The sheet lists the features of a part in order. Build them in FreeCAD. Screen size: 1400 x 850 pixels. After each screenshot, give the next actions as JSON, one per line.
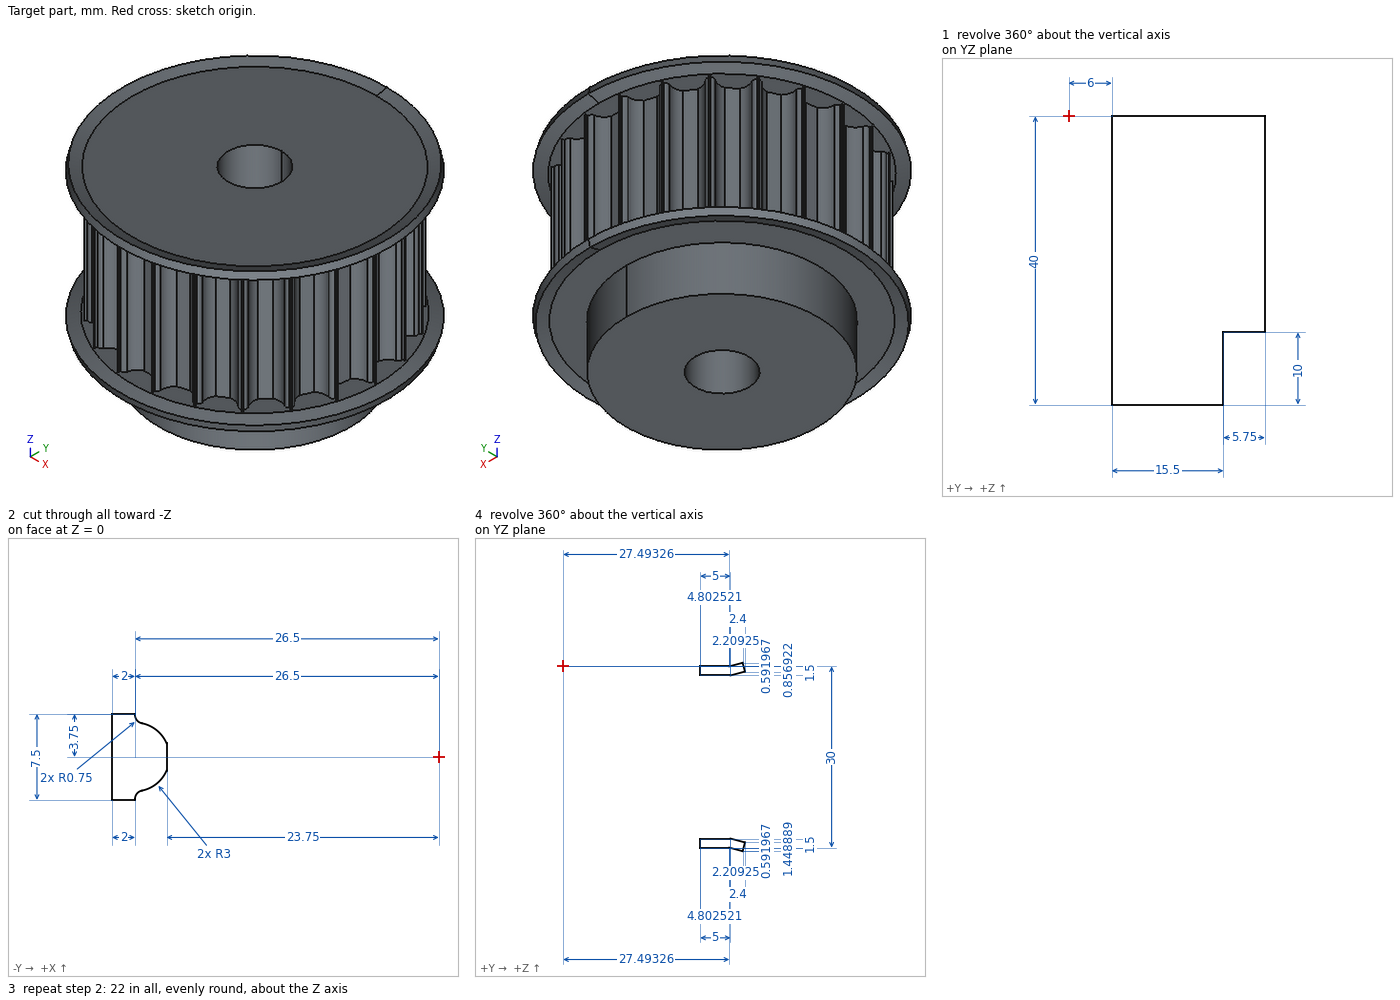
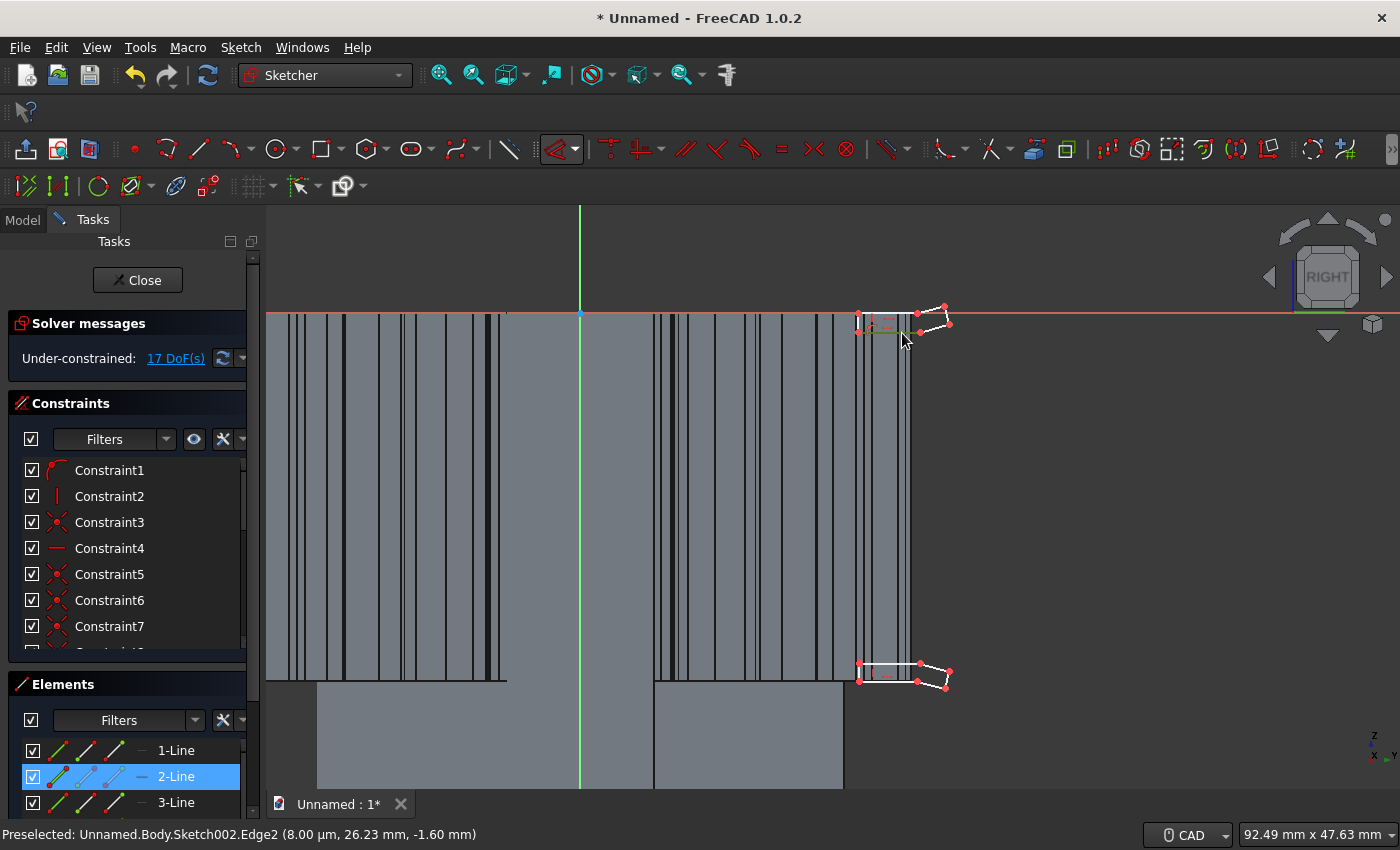
{"action": "left_click", "coordinate": [578, 150]}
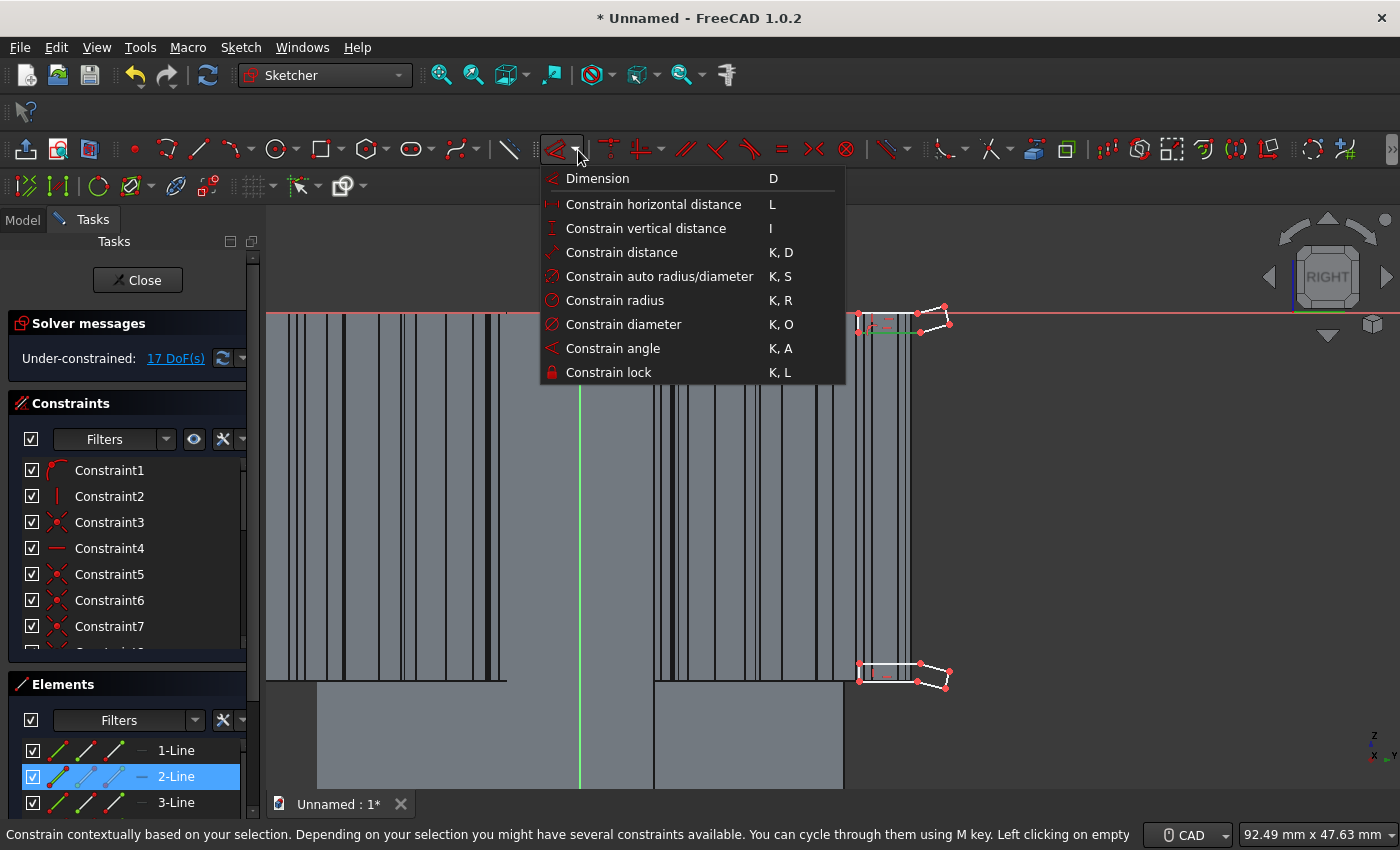
{"action": "left_click", "coordinate": [693, 204]}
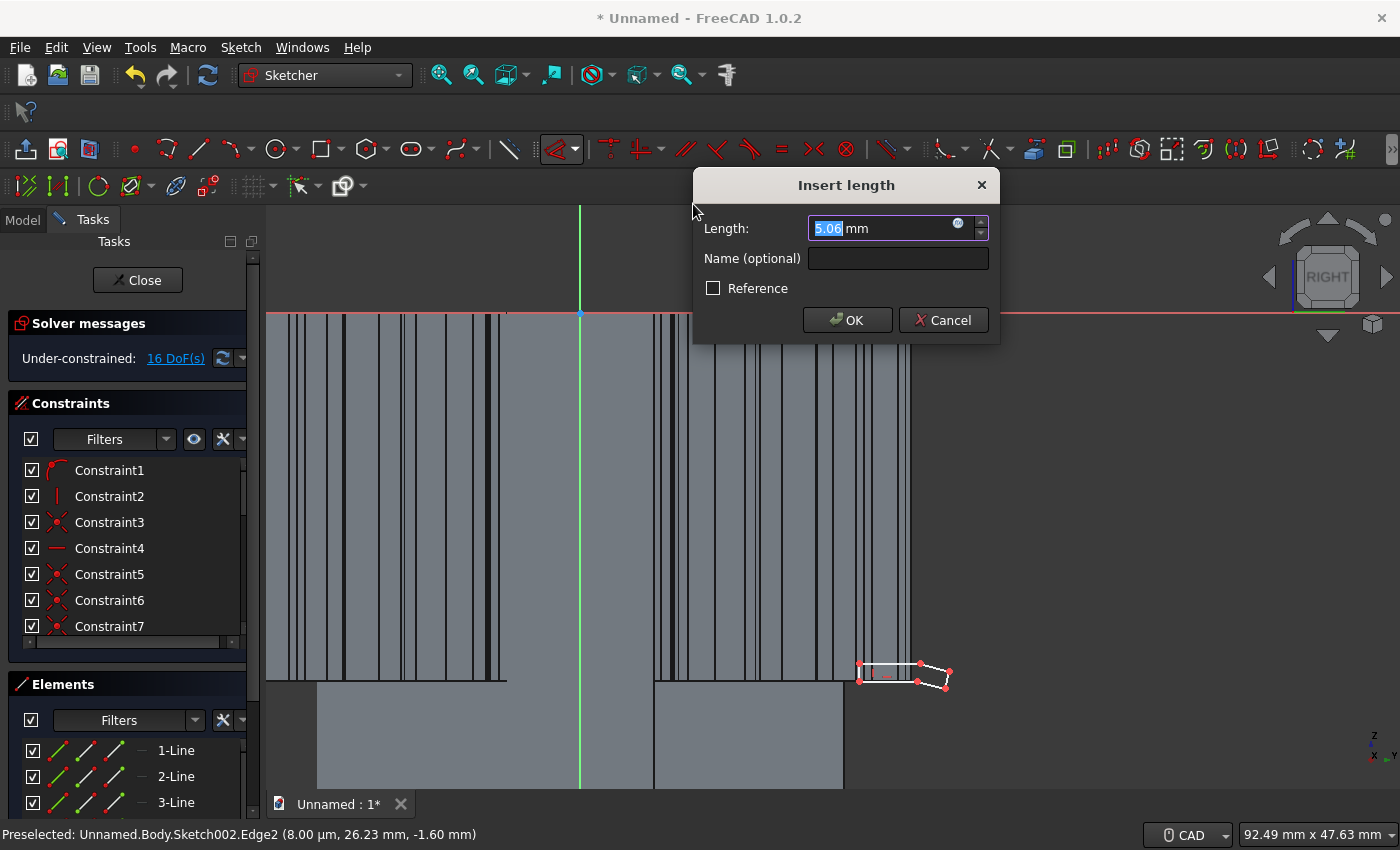
{"action": "type", "text": "5"}
{"action": "key", "text": "Return"}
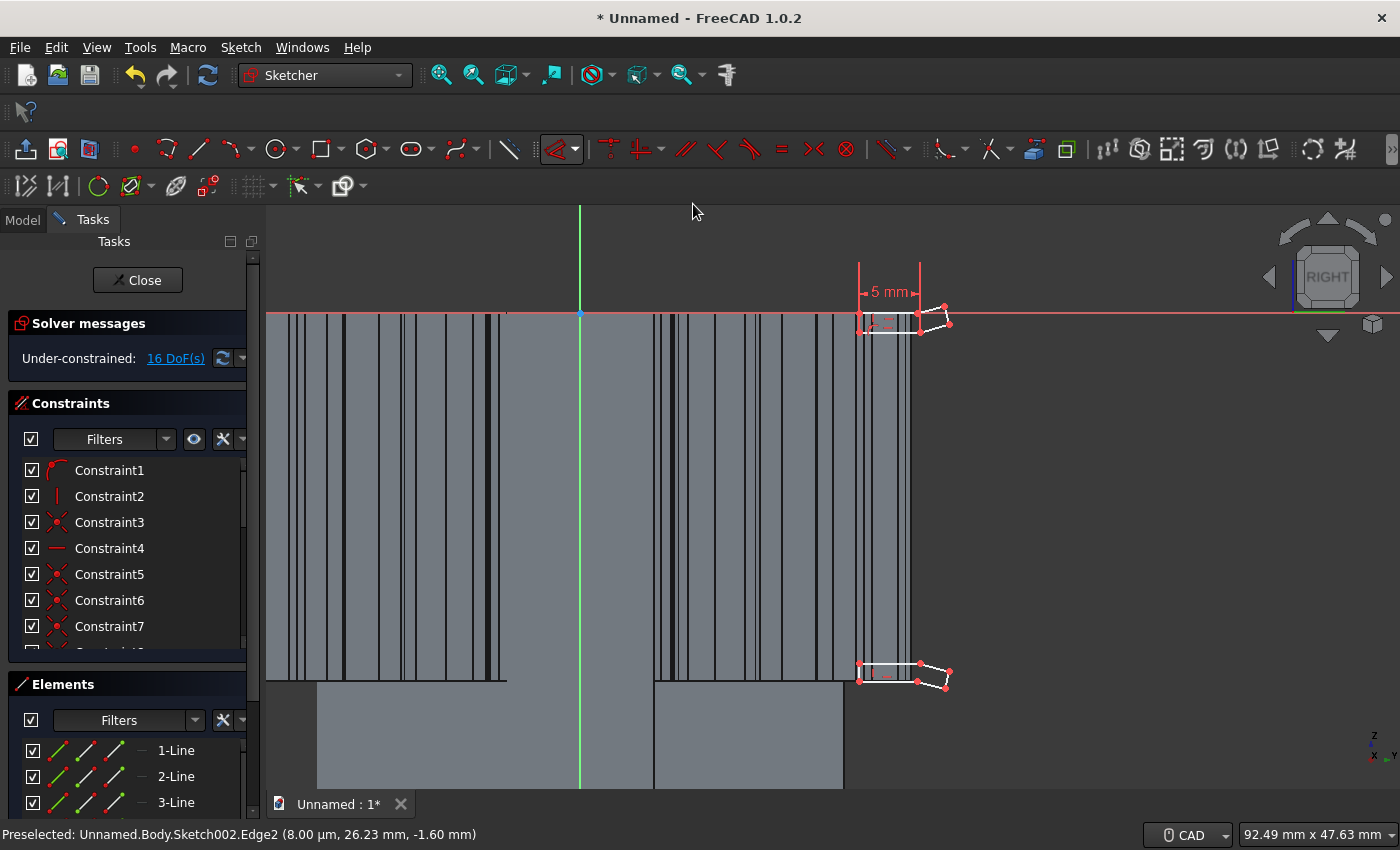
{"action": "left_click", "coordinate": [902, 664]}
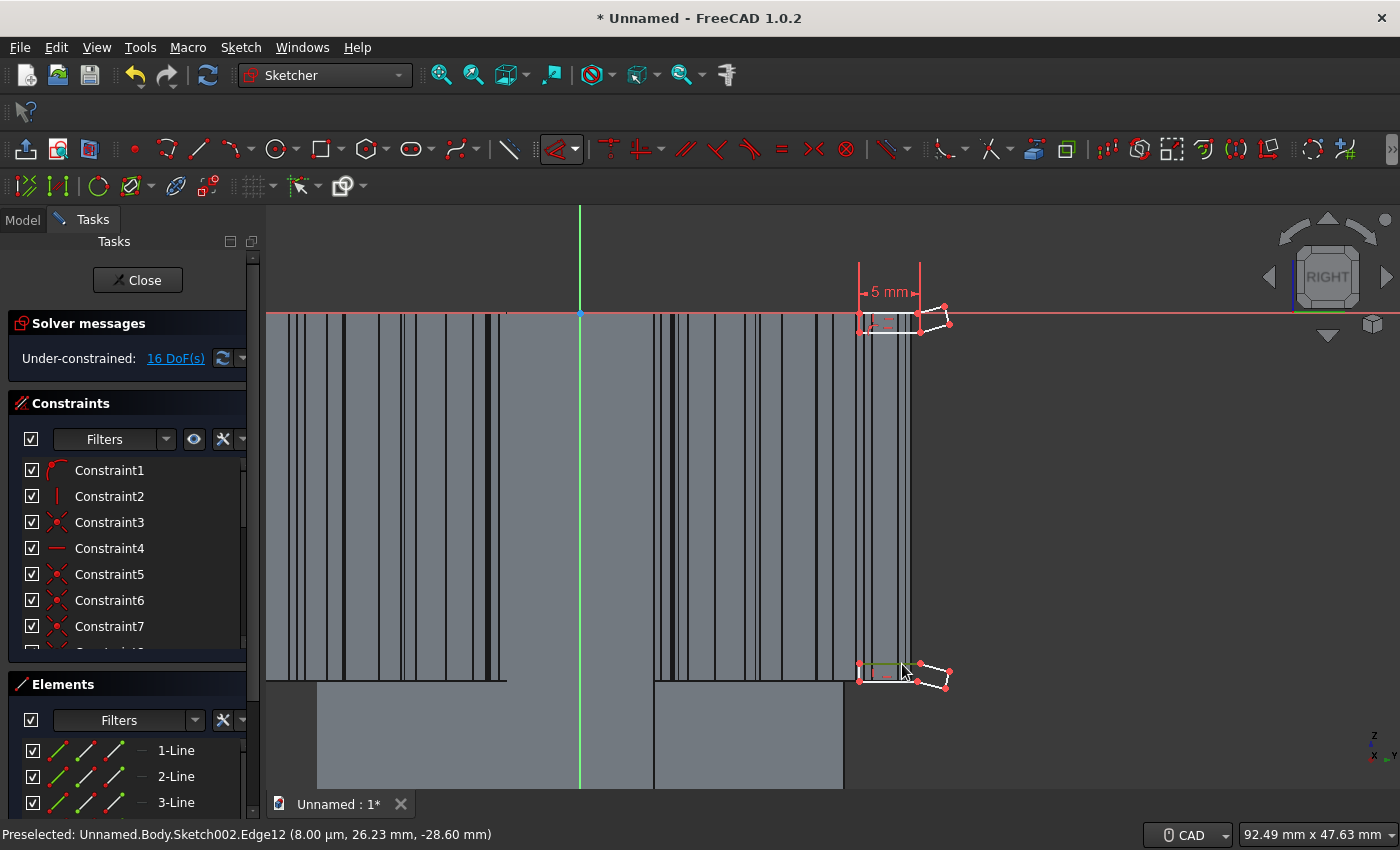
{"action": "key", "text": "l"}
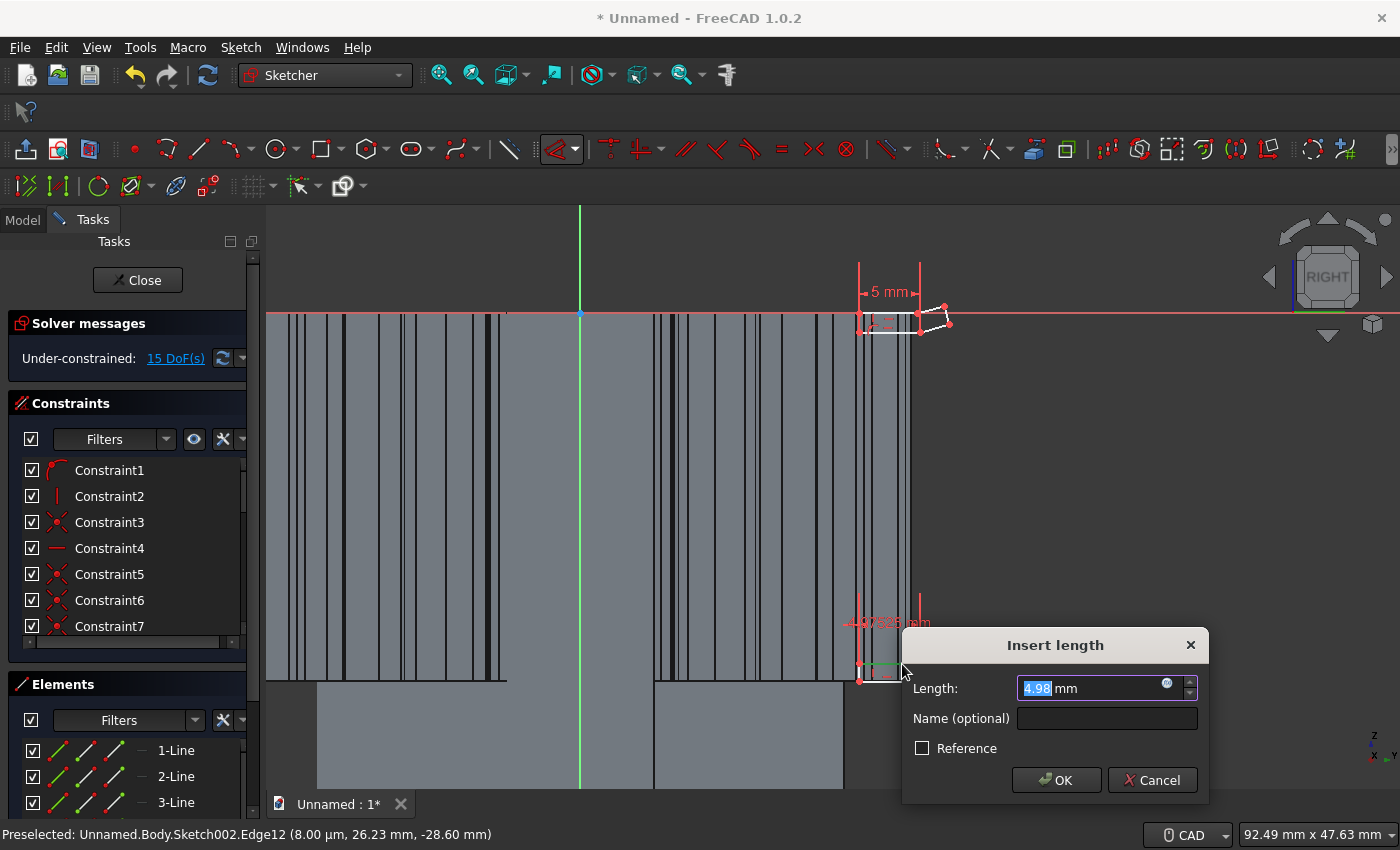
{"action": "type", "text": "5"}
{"action": "key", "text": "Return"}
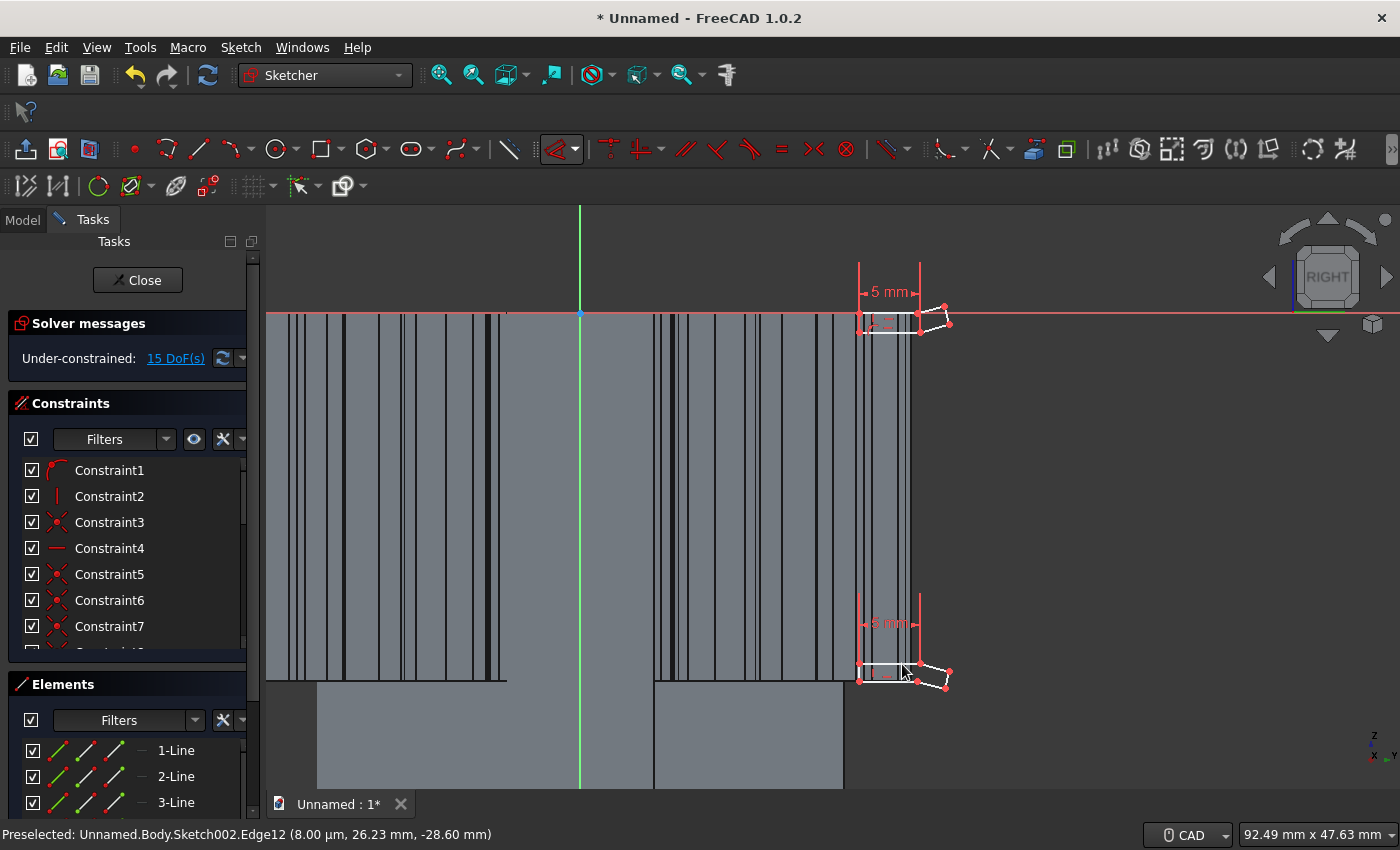
{"action": "scroll", "coordinate": [859, 323], "scroll_direction": "up", "scroll_amount": 4}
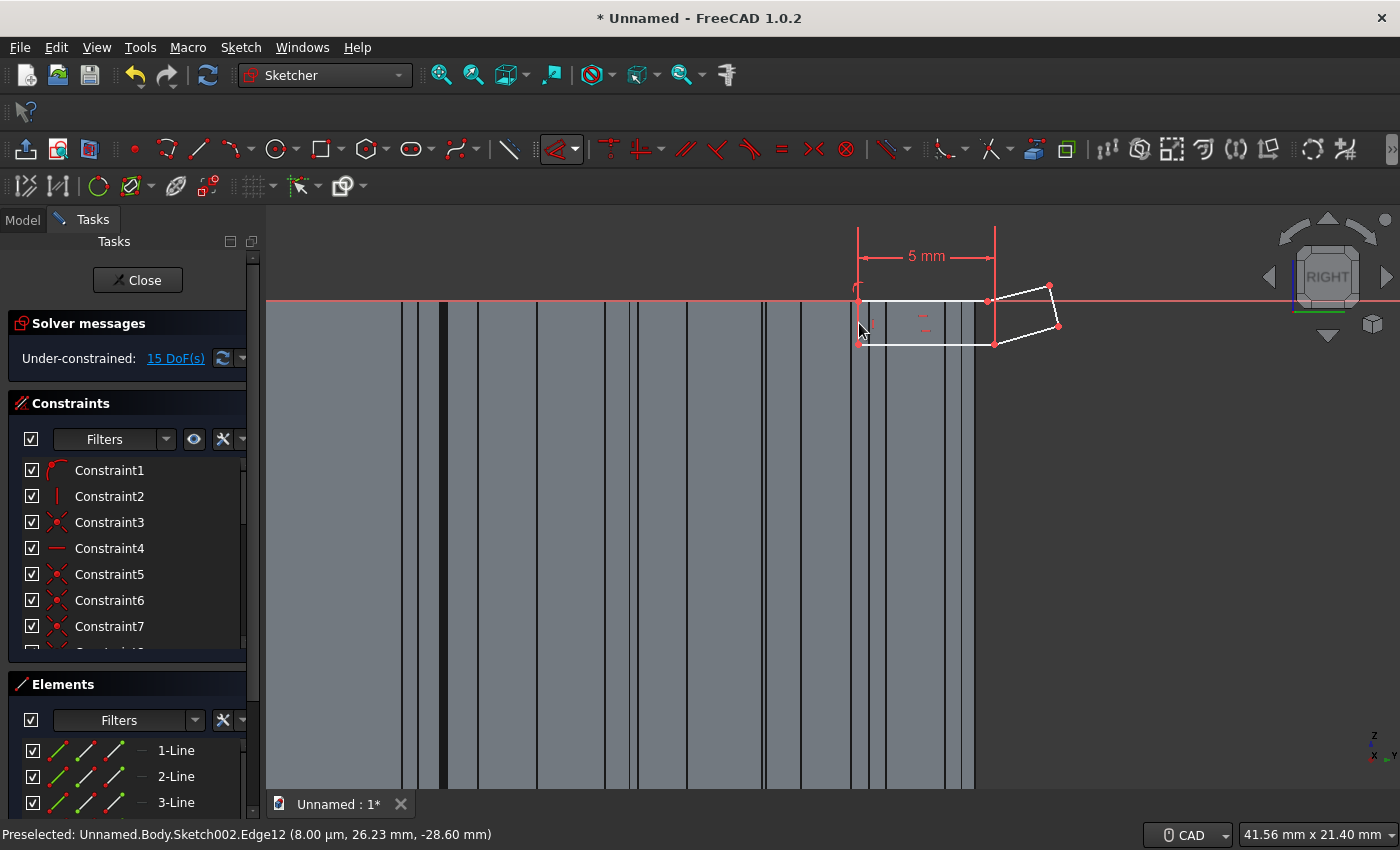
{"action": "left_click", "coordinate": [858, 323]}